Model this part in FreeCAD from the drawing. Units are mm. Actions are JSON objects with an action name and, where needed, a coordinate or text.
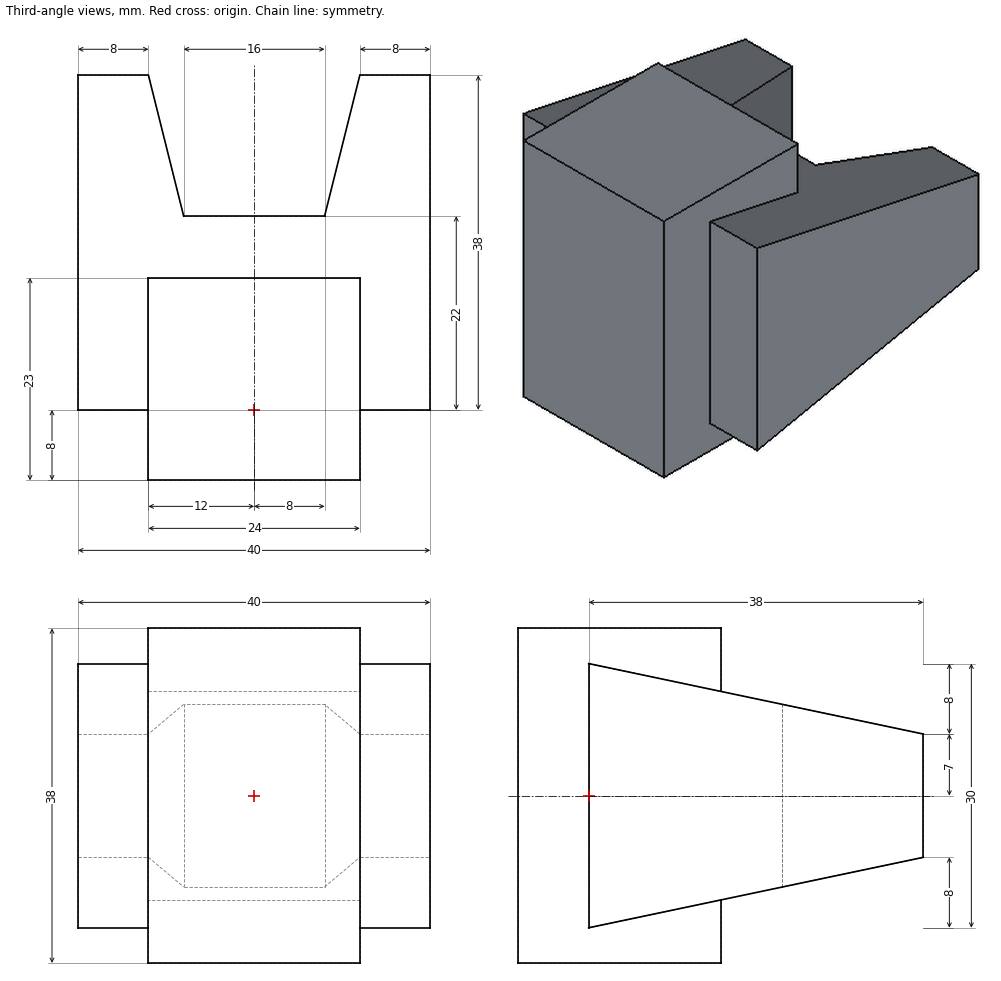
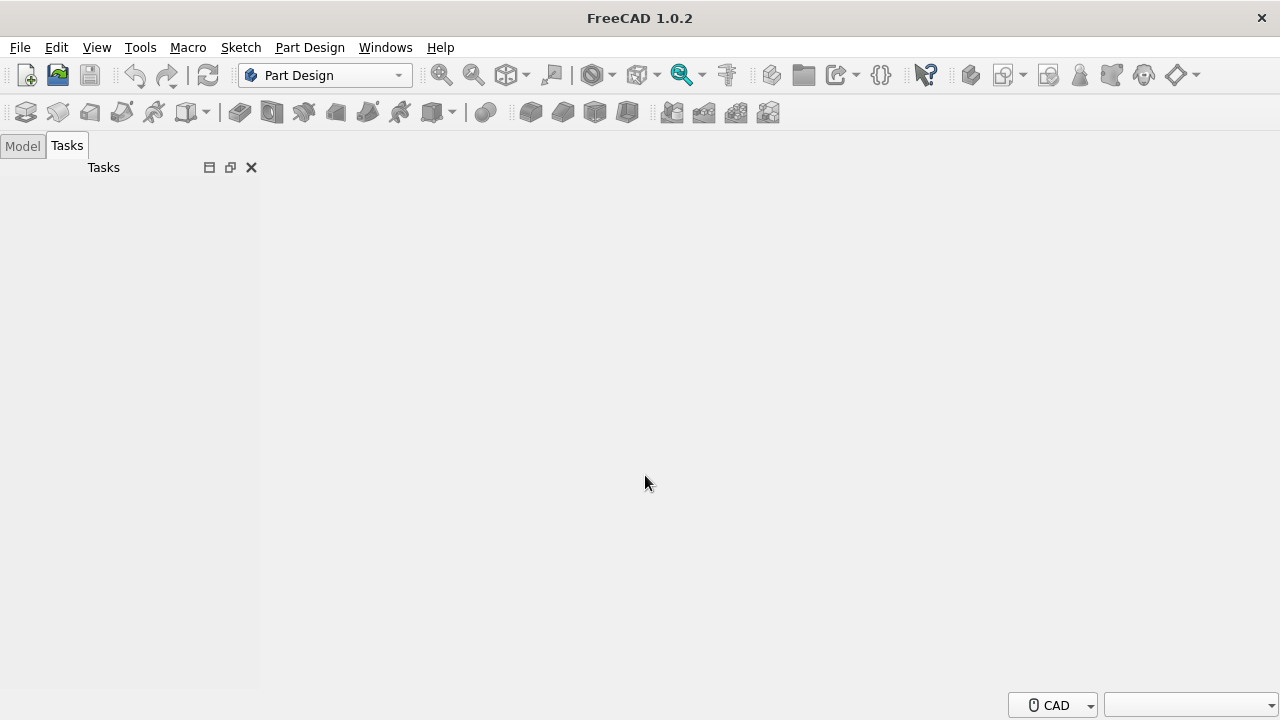
{"action": "left_click", "coordinate": [26, 76]}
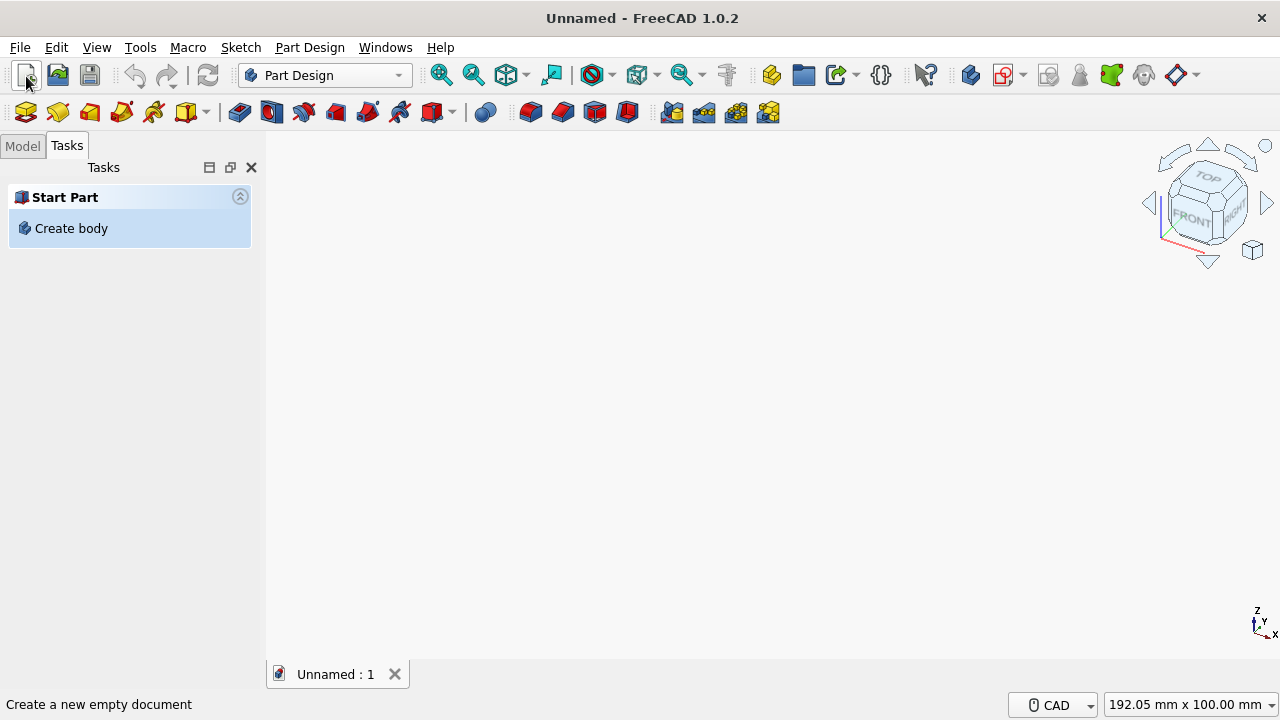
{"action": "left_click", "coordinate": [1004, 76]}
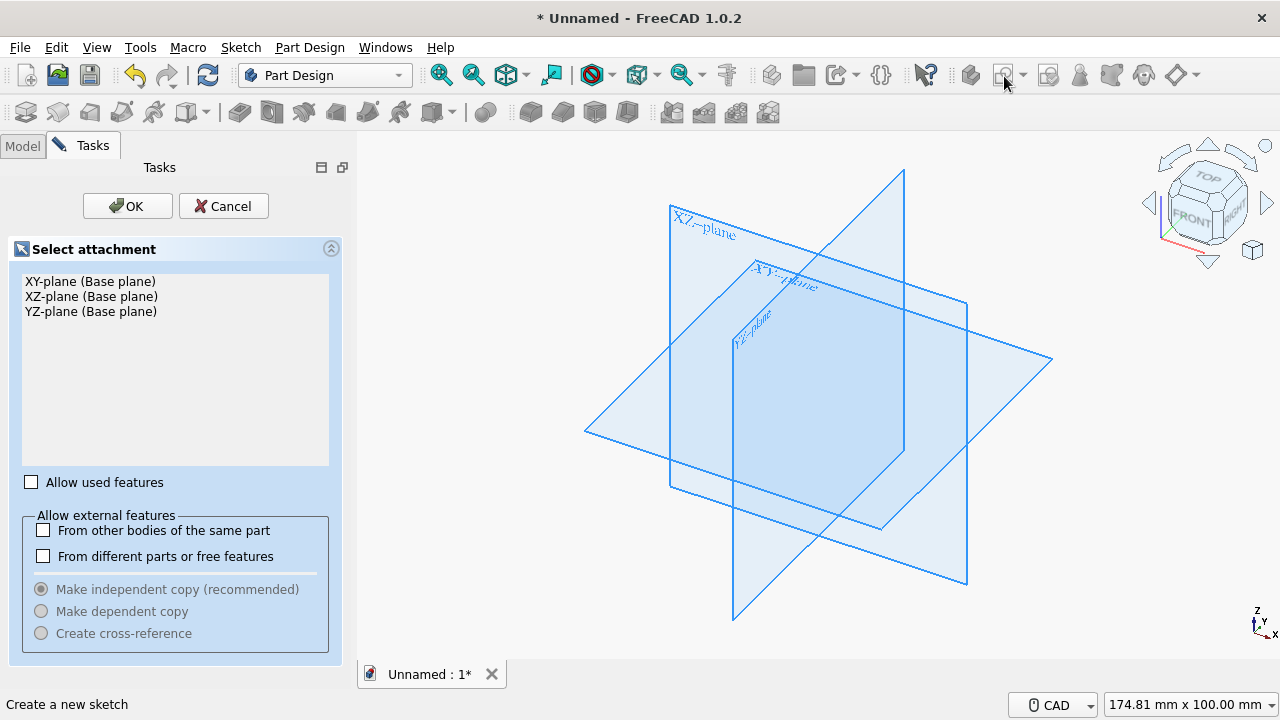
{"action": "left_click", "coordinate": [82, 282]}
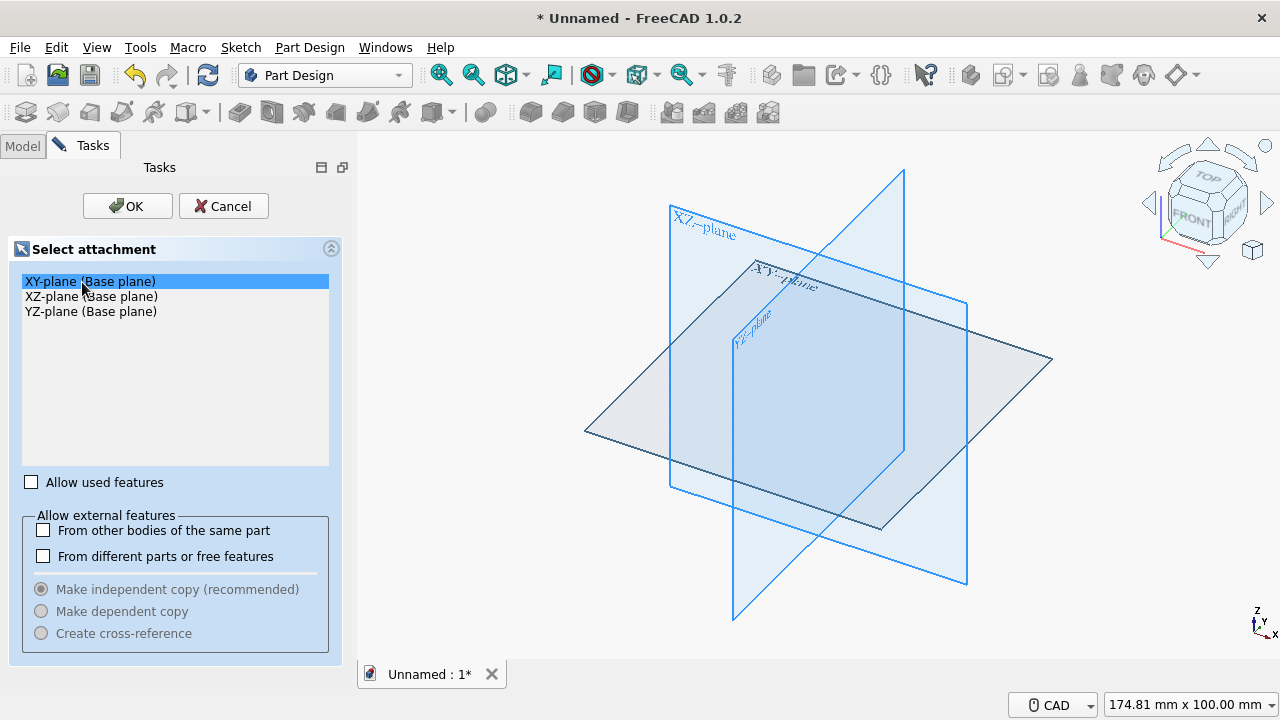
{"action": "left_click", "coordinate": [128, 206]}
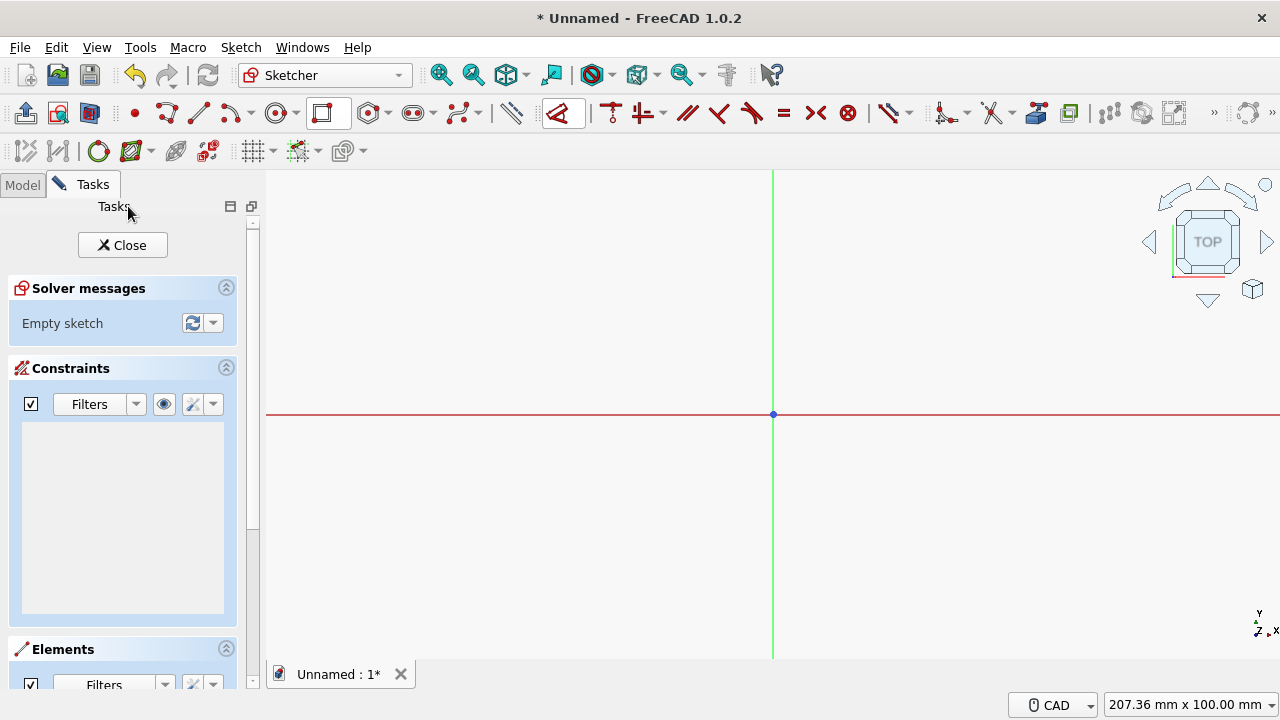
{"action": "scroll", "coordinate": [912, 198], "scroll_direction": "up", "scroll_amount": 2}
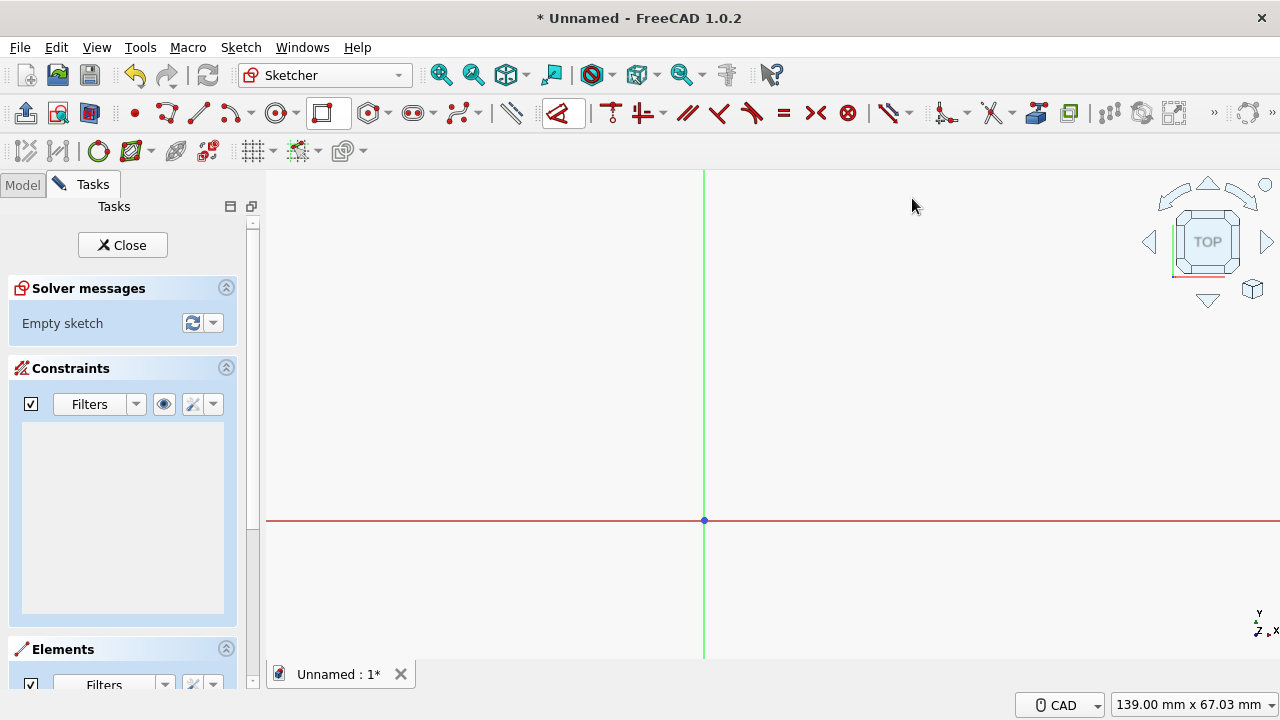
{"action": "left_click", "coordinate": [168, 114]}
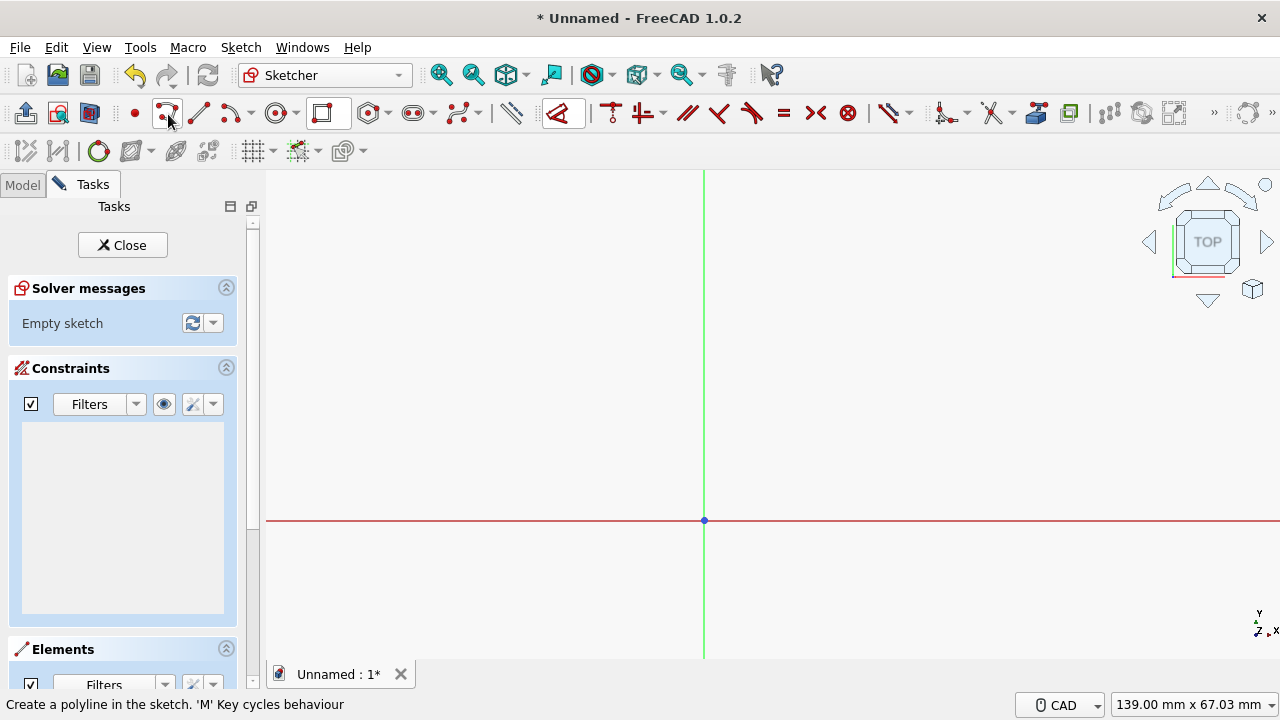
{"action": "left_click", "coordinate": [558, 521]}
{"action": "left_click", "coordinate": [850, 512]}
{"action": "left_click", "coordinate": [850, 244]}
{"action": "left_click", "coordinate": [792, 244]}
{"action": "left_click", "coordinate": [763, 360]}
{"action": "left_click", "coordinate": [646, 360]}
{"action": "left_click", "coordinate": [617, 244]}
{"action": "left_click", "coordinate": [558, 244]}
{"action": "left_click", "coordinate": [558, 521]}
{"action": "key", "text": "Escape"}
{"action": "key", "text": "Escape"}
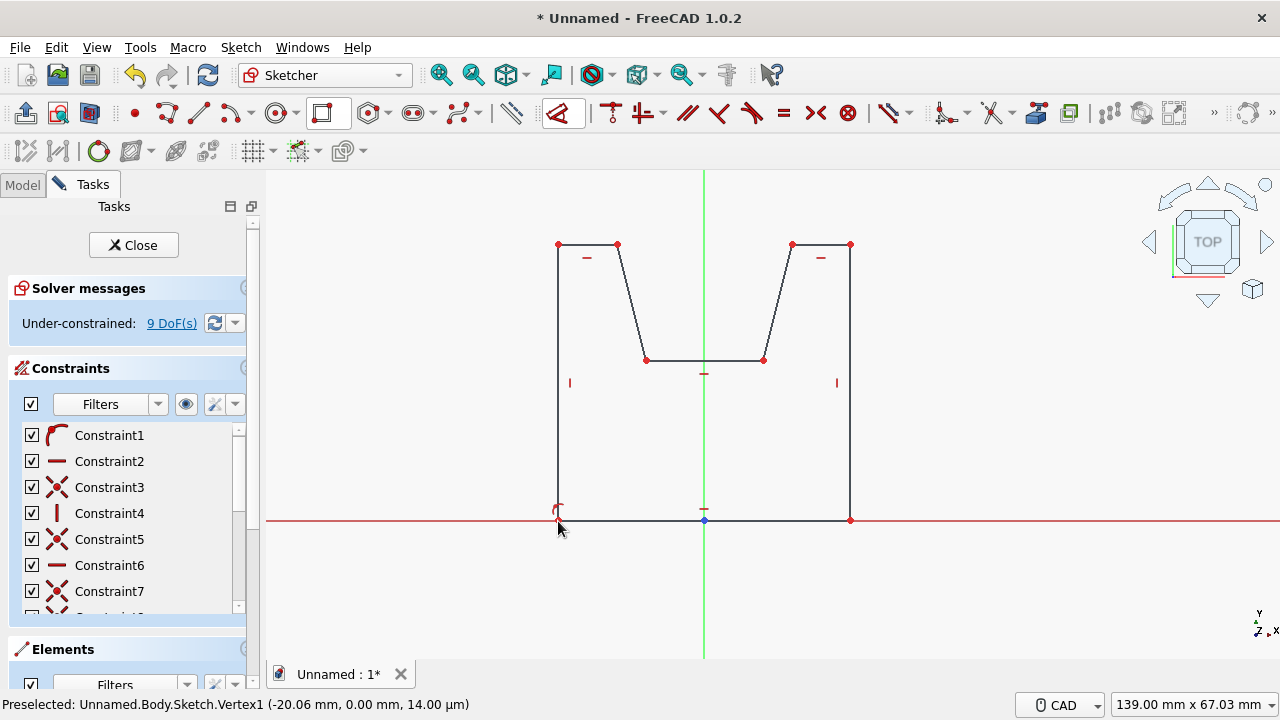
{"action": "left_click", "coordinate": [792, 245]}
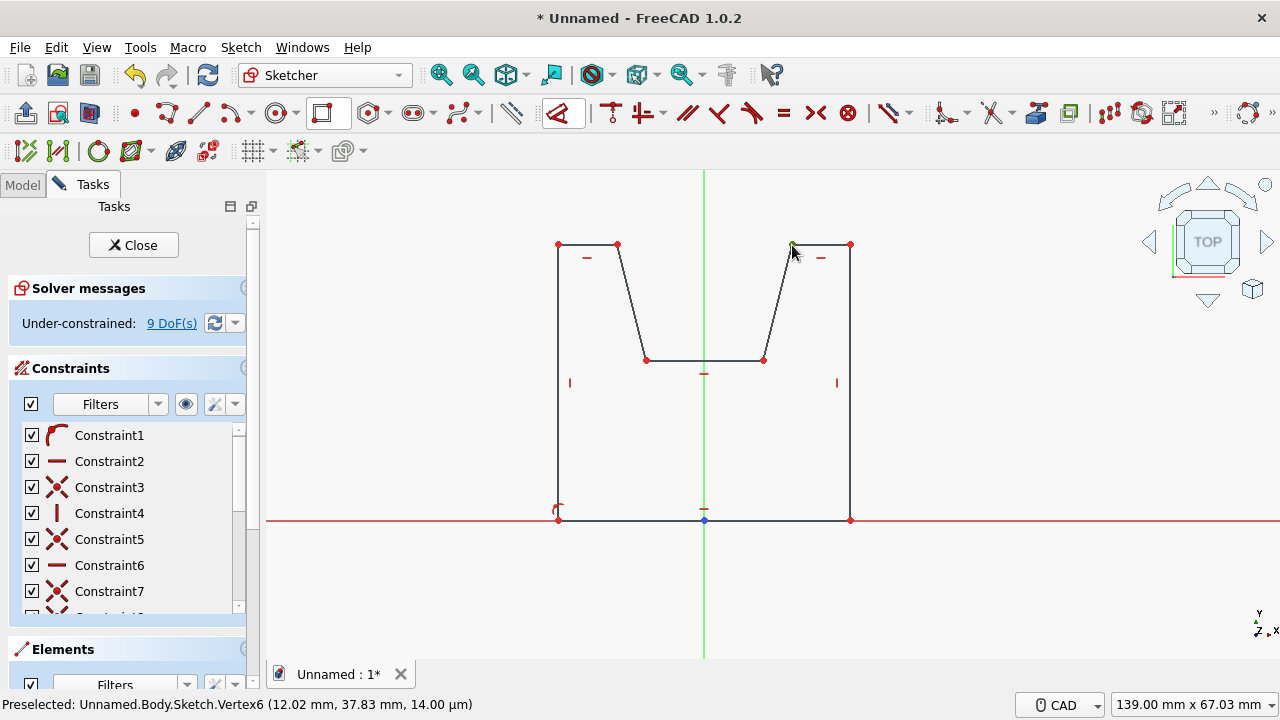
{"action": "left_click", "coordinate": [617, 245]}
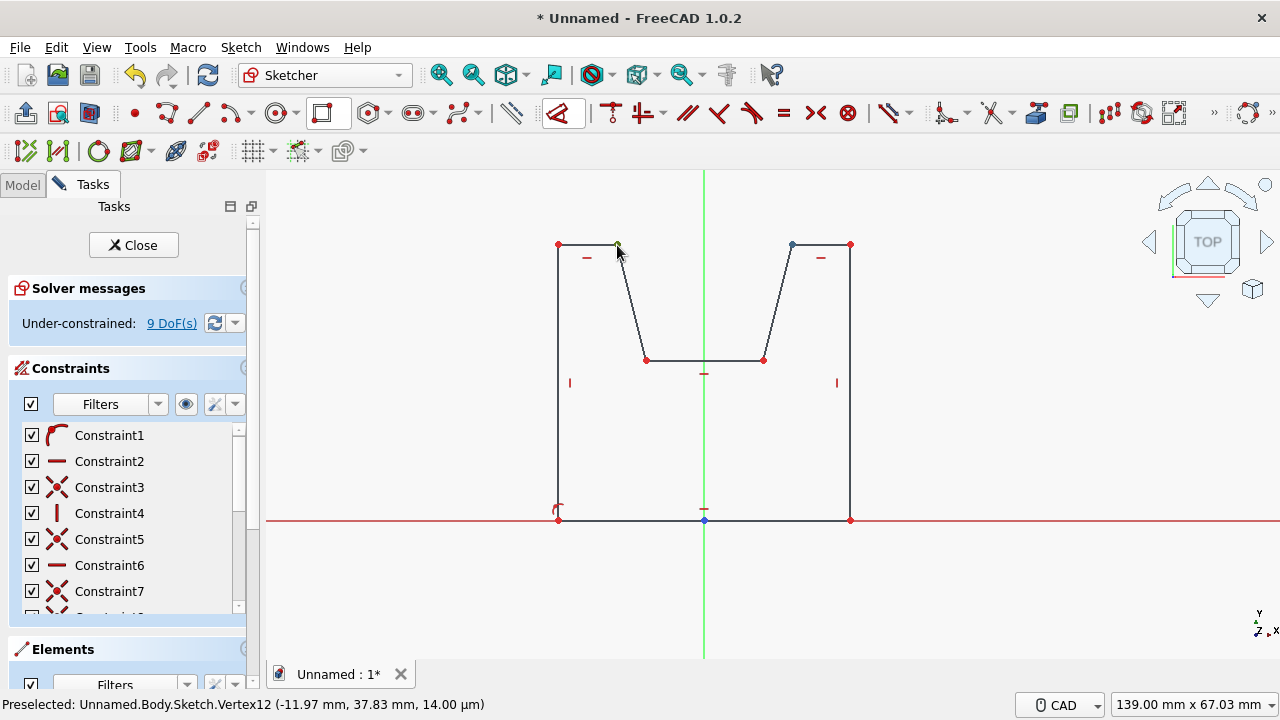
{"action": "left_click", "coordinate": [704, 600]}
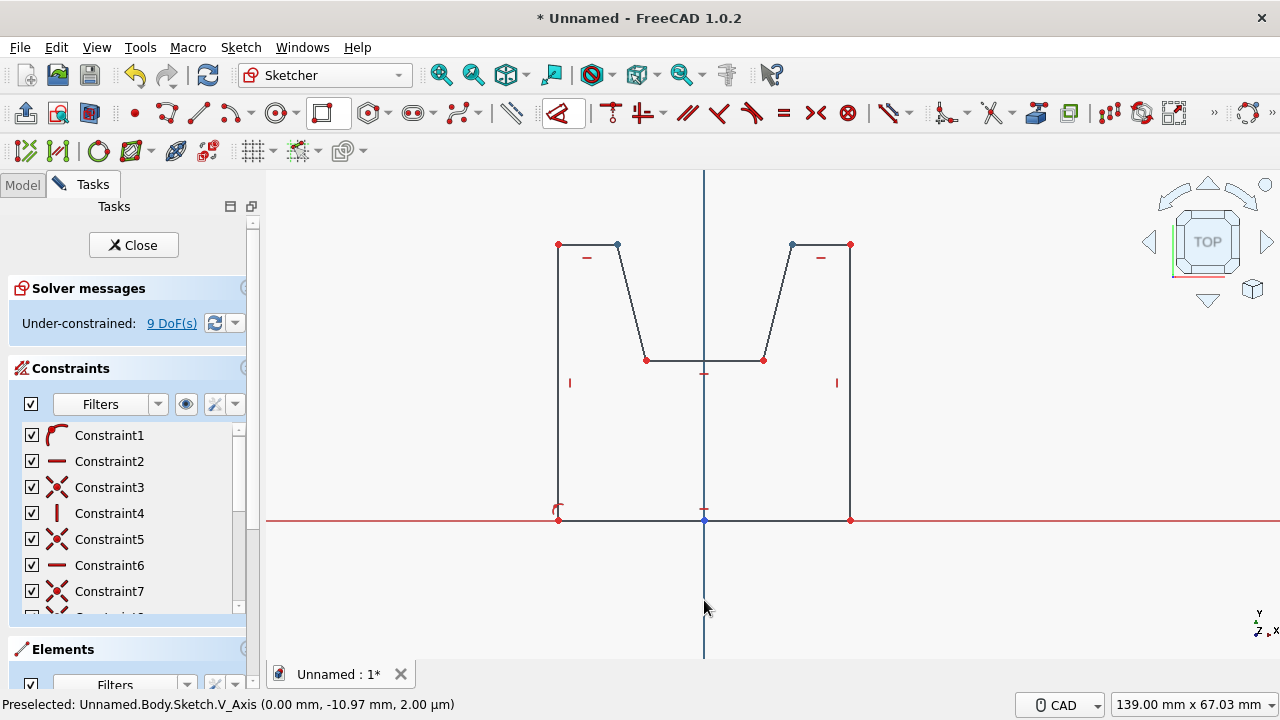
{"action": "left_click", "coordinate": [816, 114]}